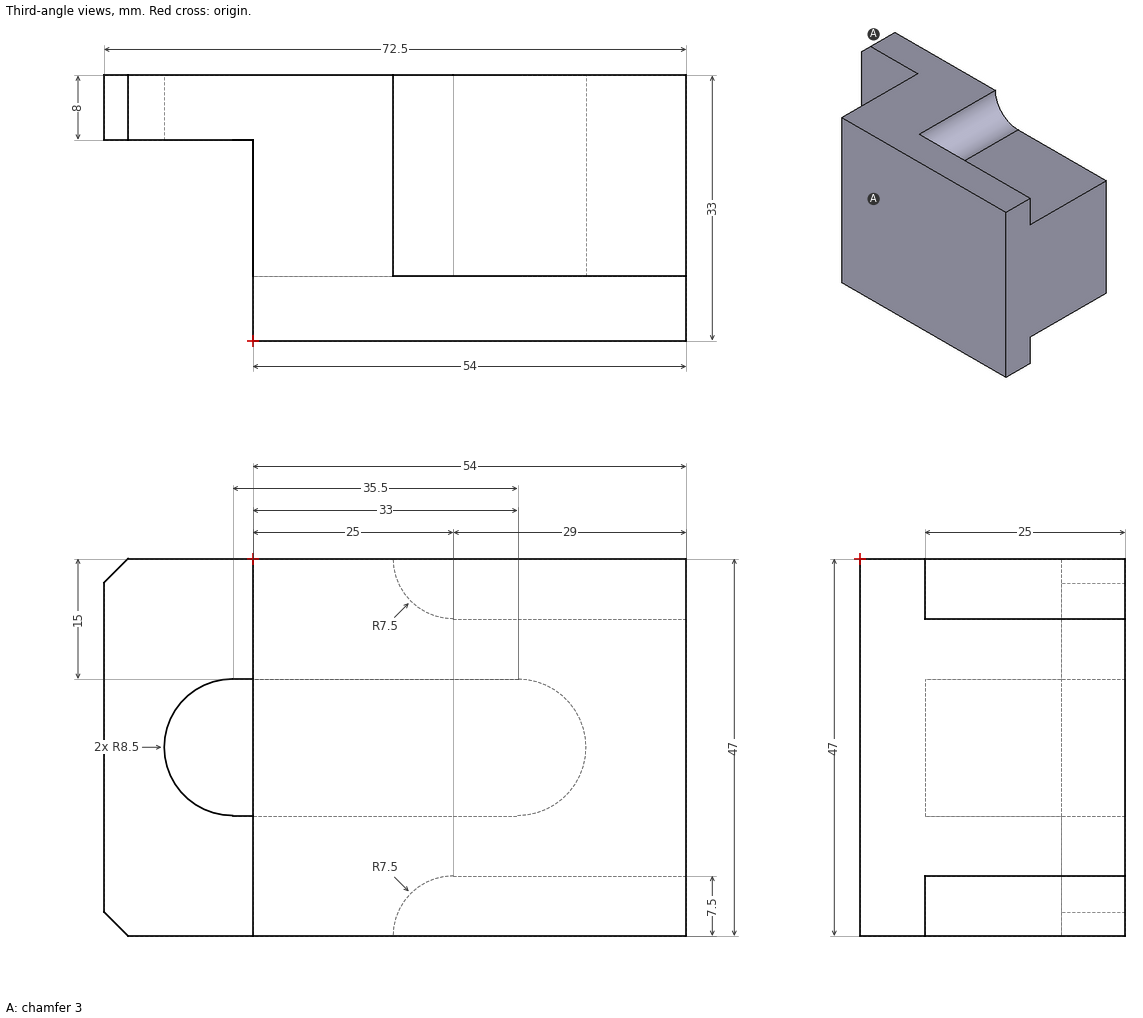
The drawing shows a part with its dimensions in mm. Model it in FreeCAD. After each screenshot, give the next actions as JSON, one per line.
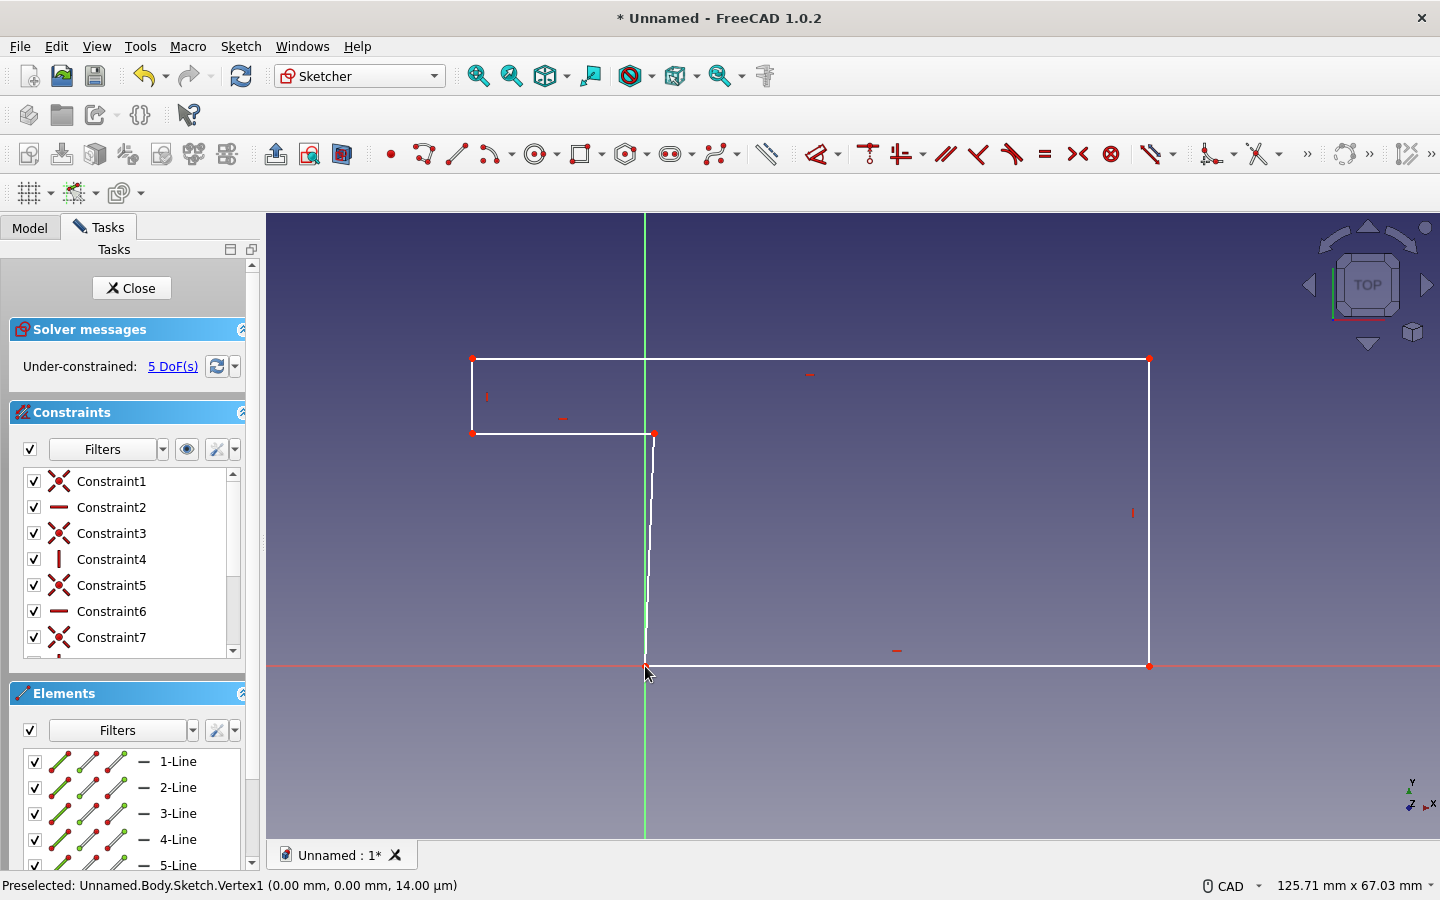
{"action": "left_click", "coordinate": [648, 597]}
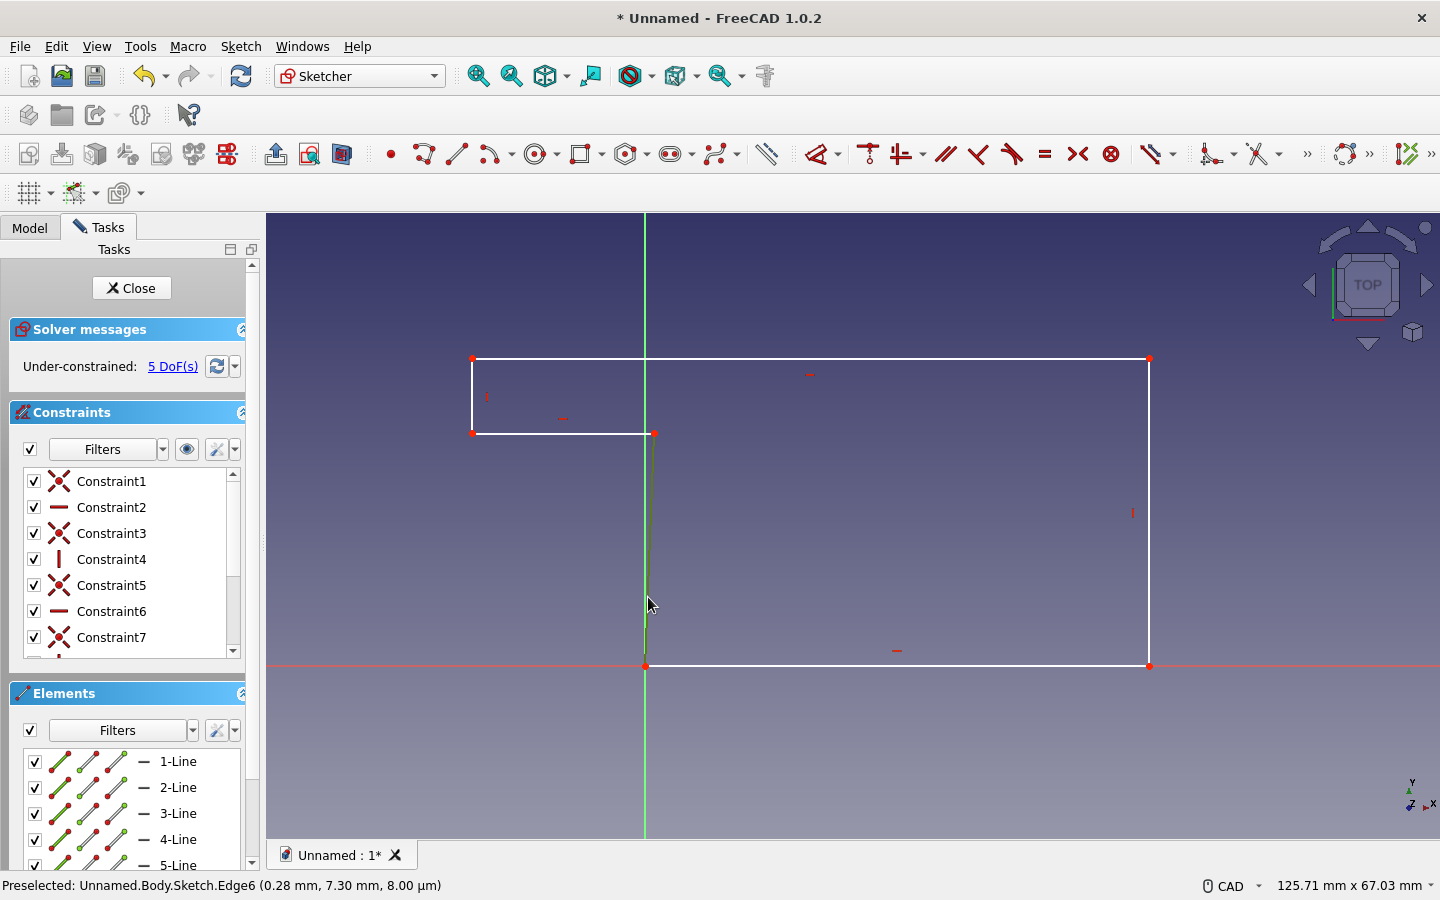
{"action": "key", "text": "v"}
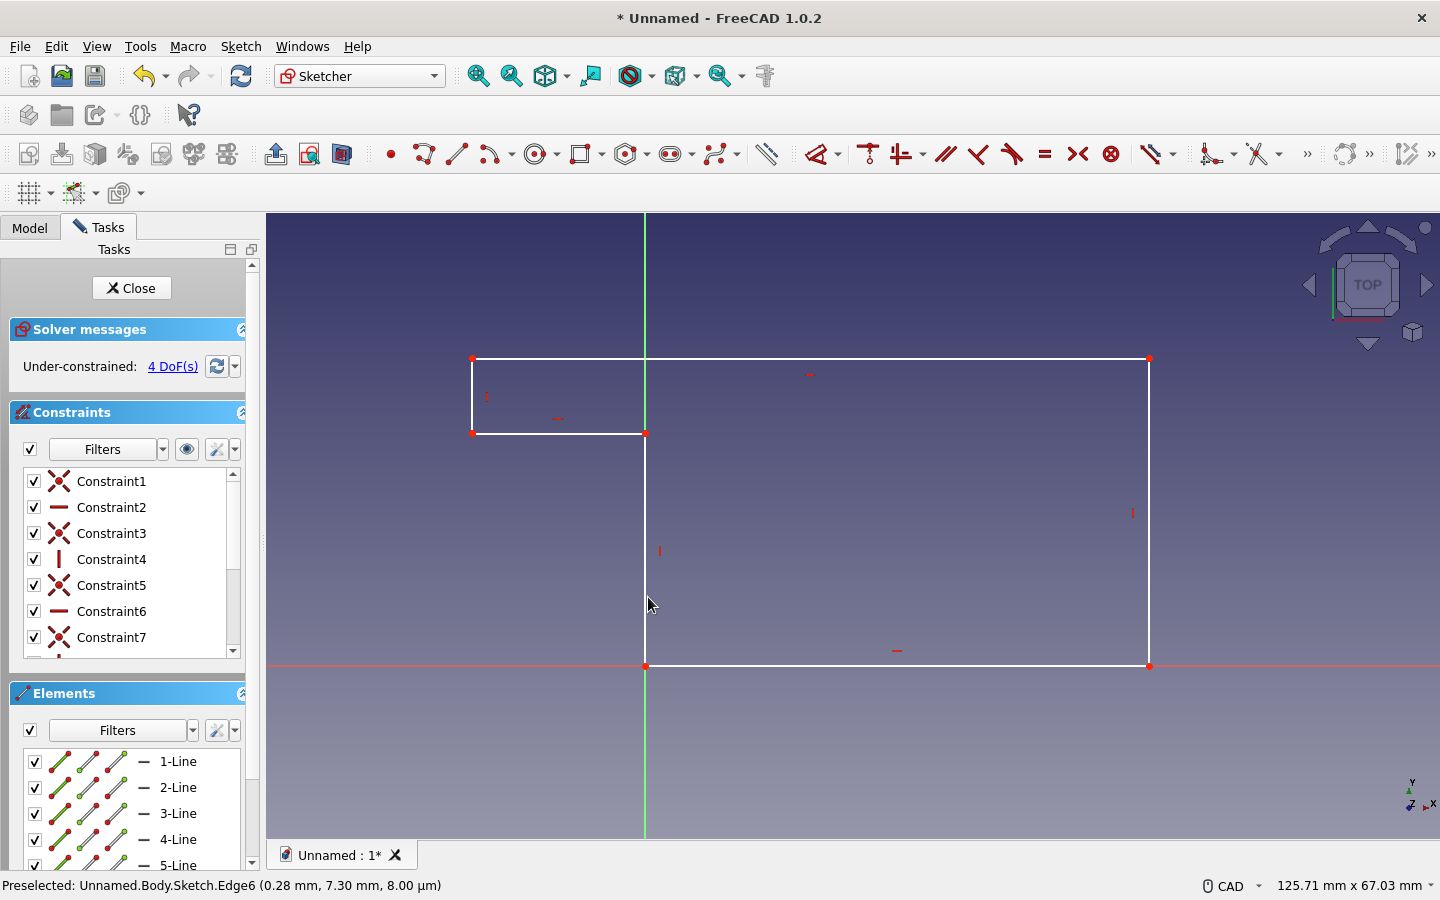
{"action": "key", "text": "d"}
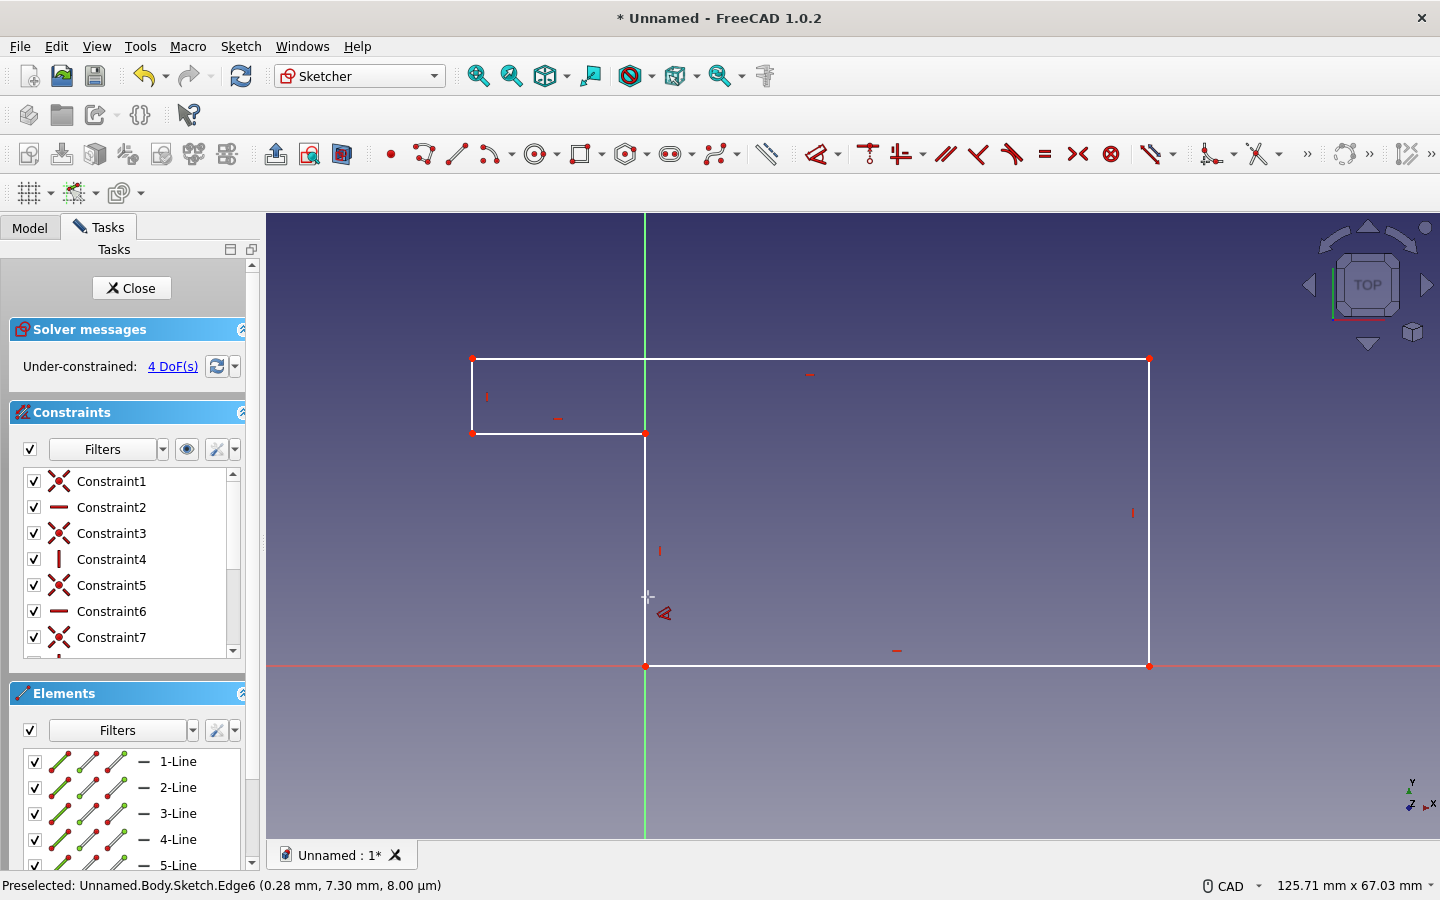
{"action": "left_click", "coordinate": [472, 382]}
{"action": "left_click", "coordinate": [438, 397]}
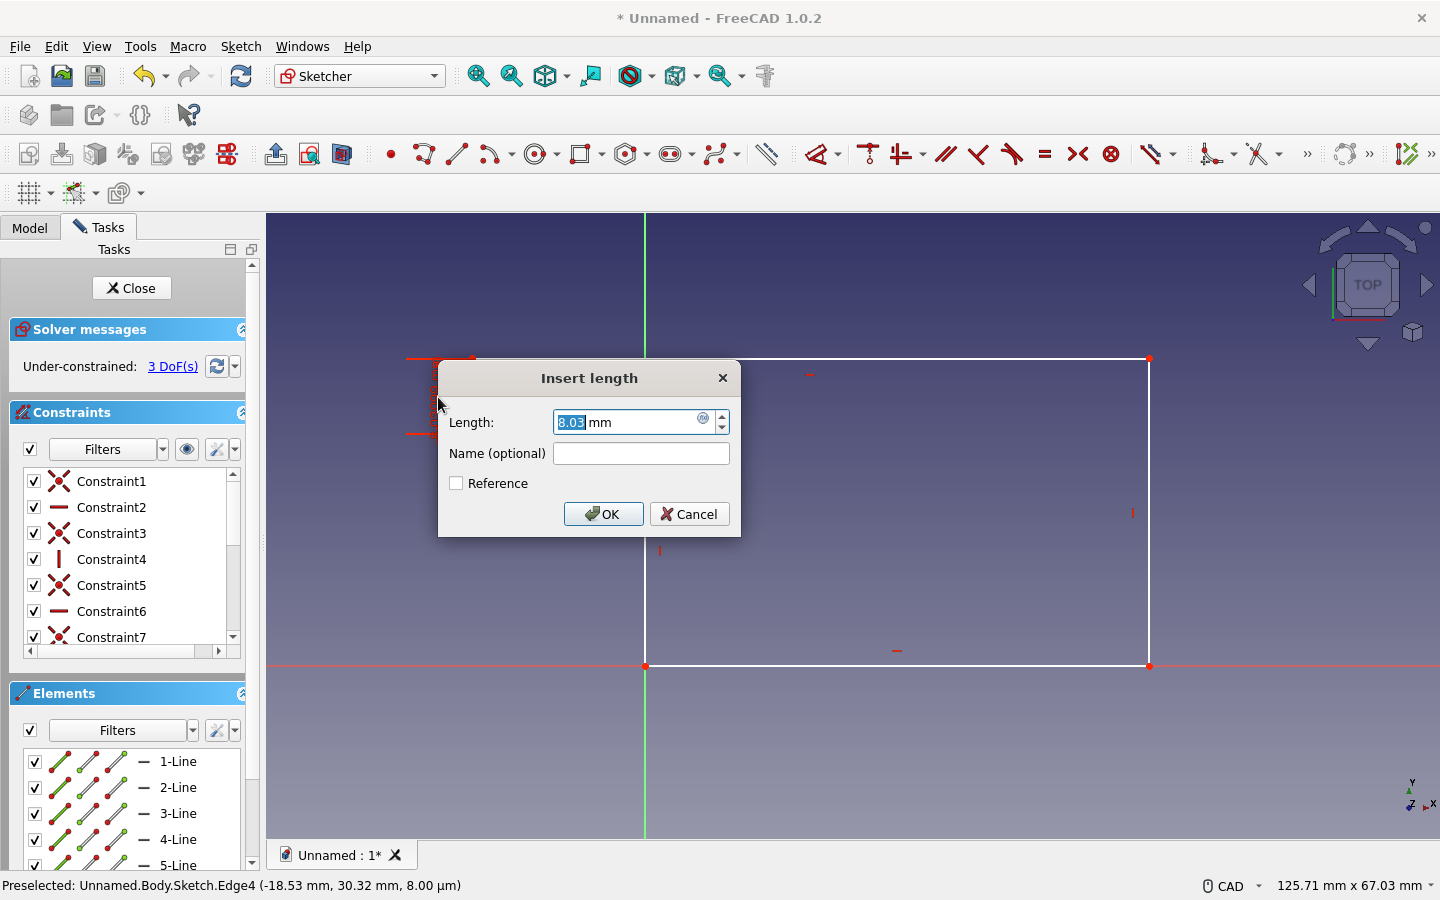
{"action": "type", "text": "8"}
{"action": "key", "text": "Return"}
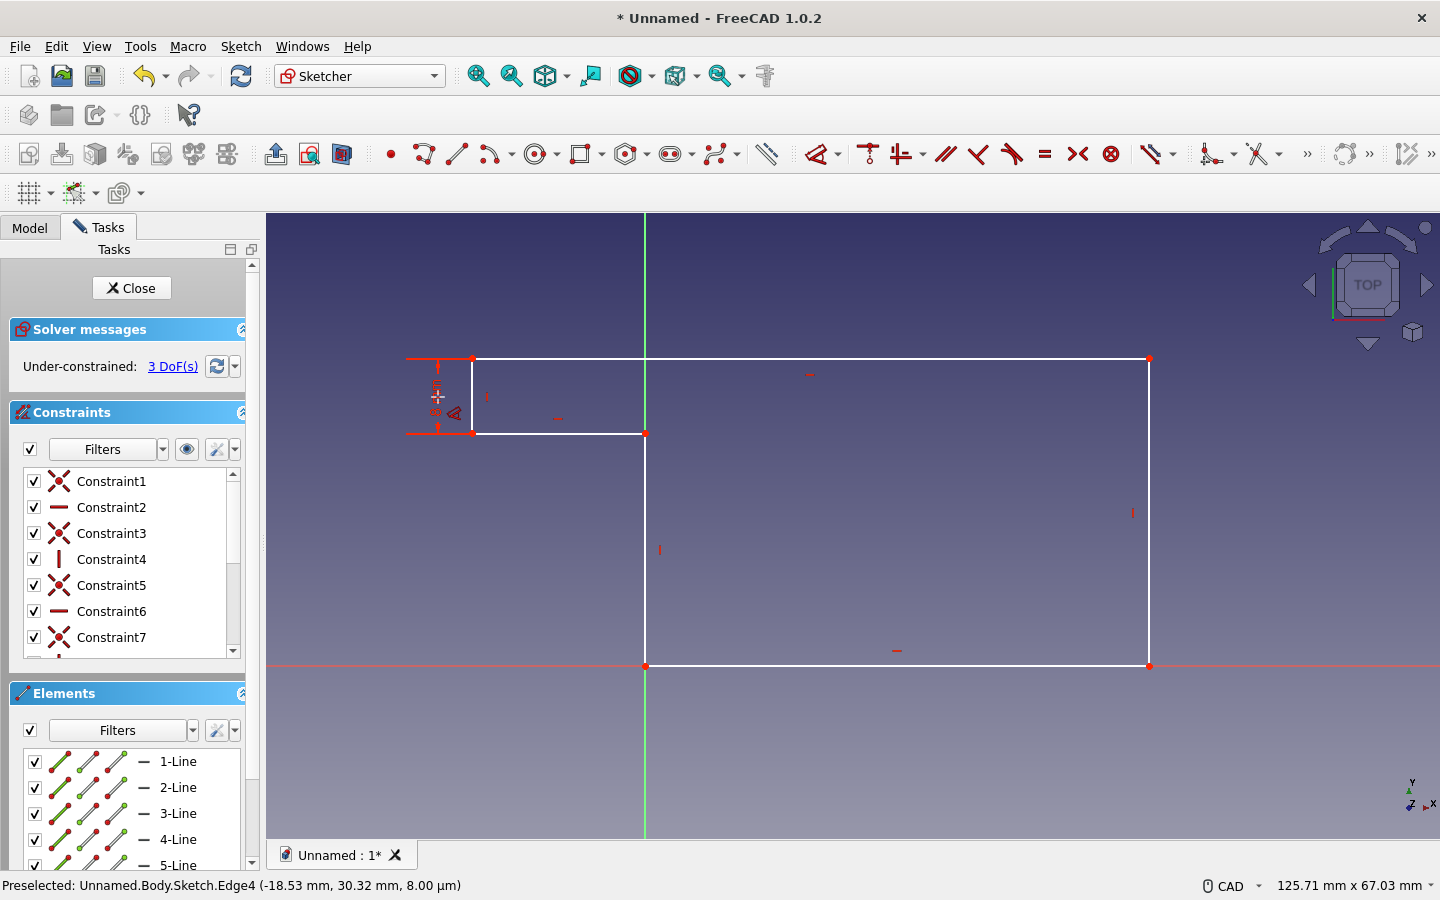
{"action": "left_click", "coordinate": [796, 666]}
{"action": "left_click", "coordinate": [897, 700]}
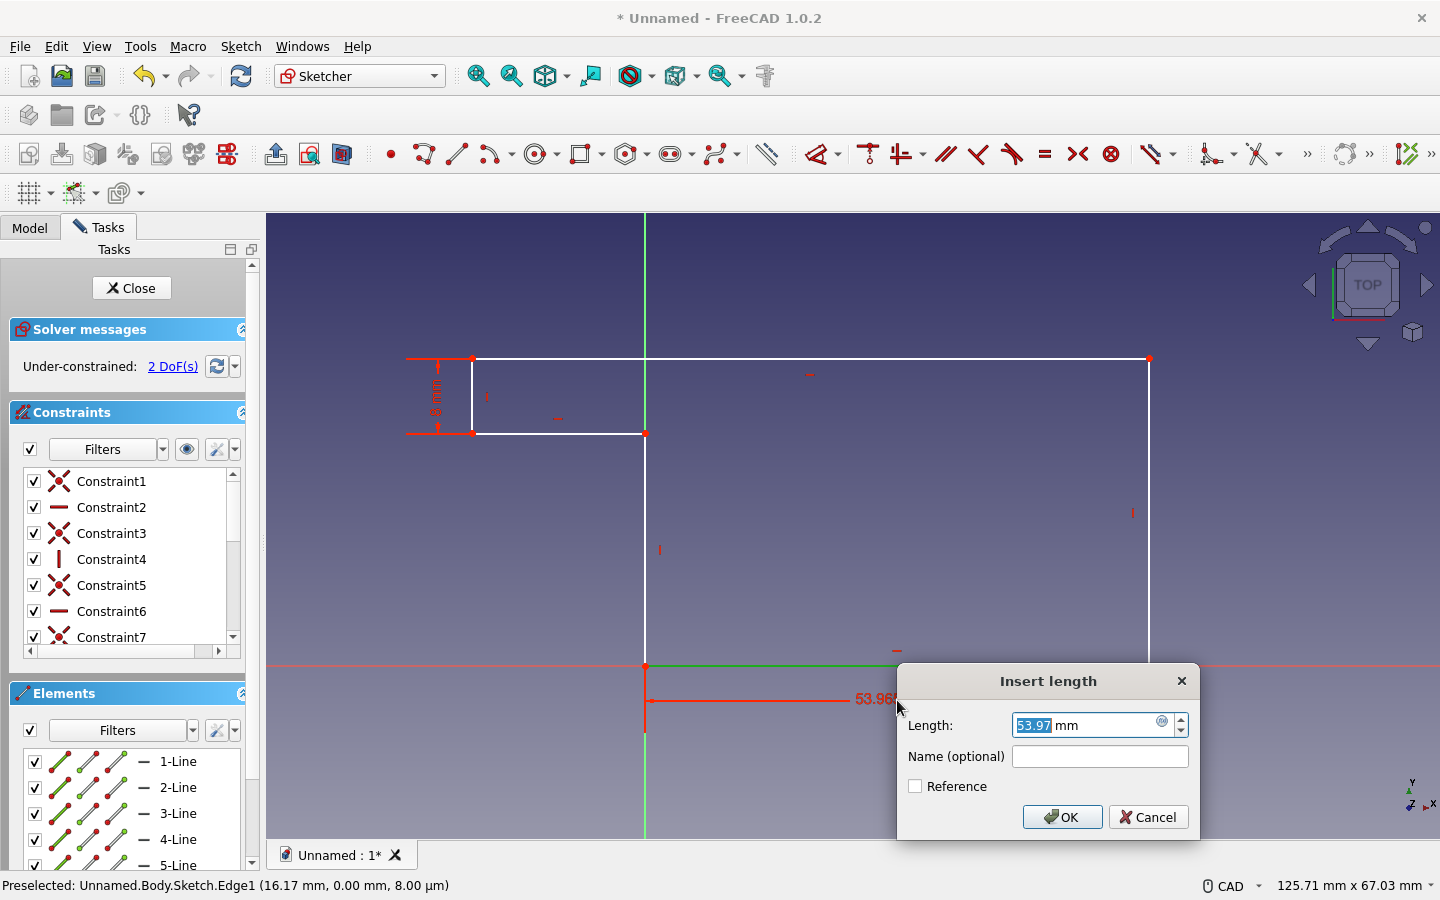
{"action": "type", "text": "54"}
{"action": "key", "text": "Return"}